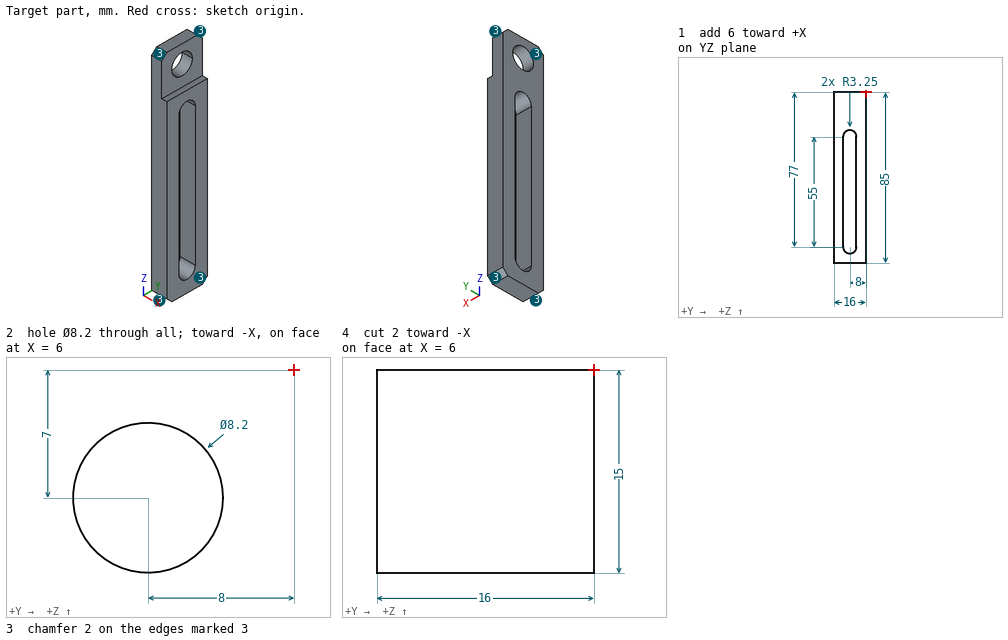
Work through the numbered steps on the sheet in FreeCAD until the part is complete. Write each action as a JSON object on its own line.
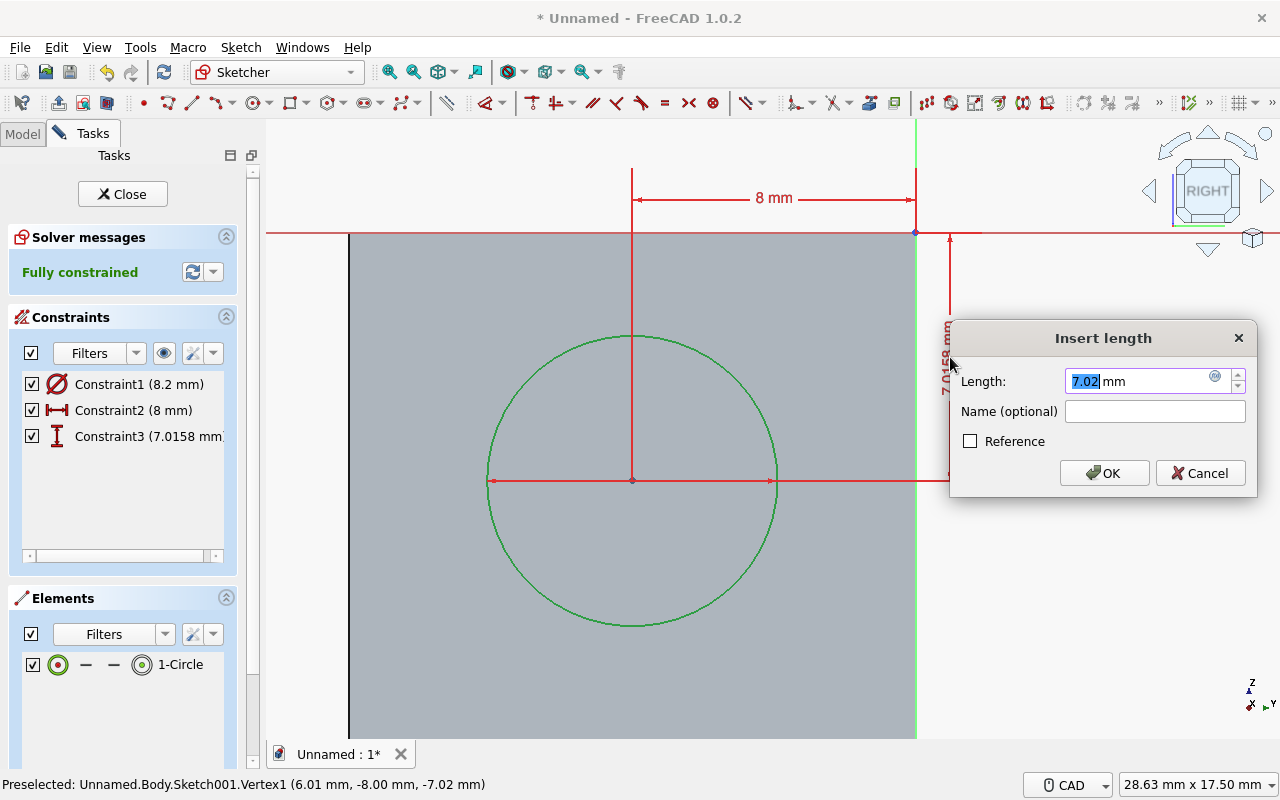
{"action": "type", "text": "7"}
{"action": "key", "text": "Return"}
{"action": "key", "text": "Escape"}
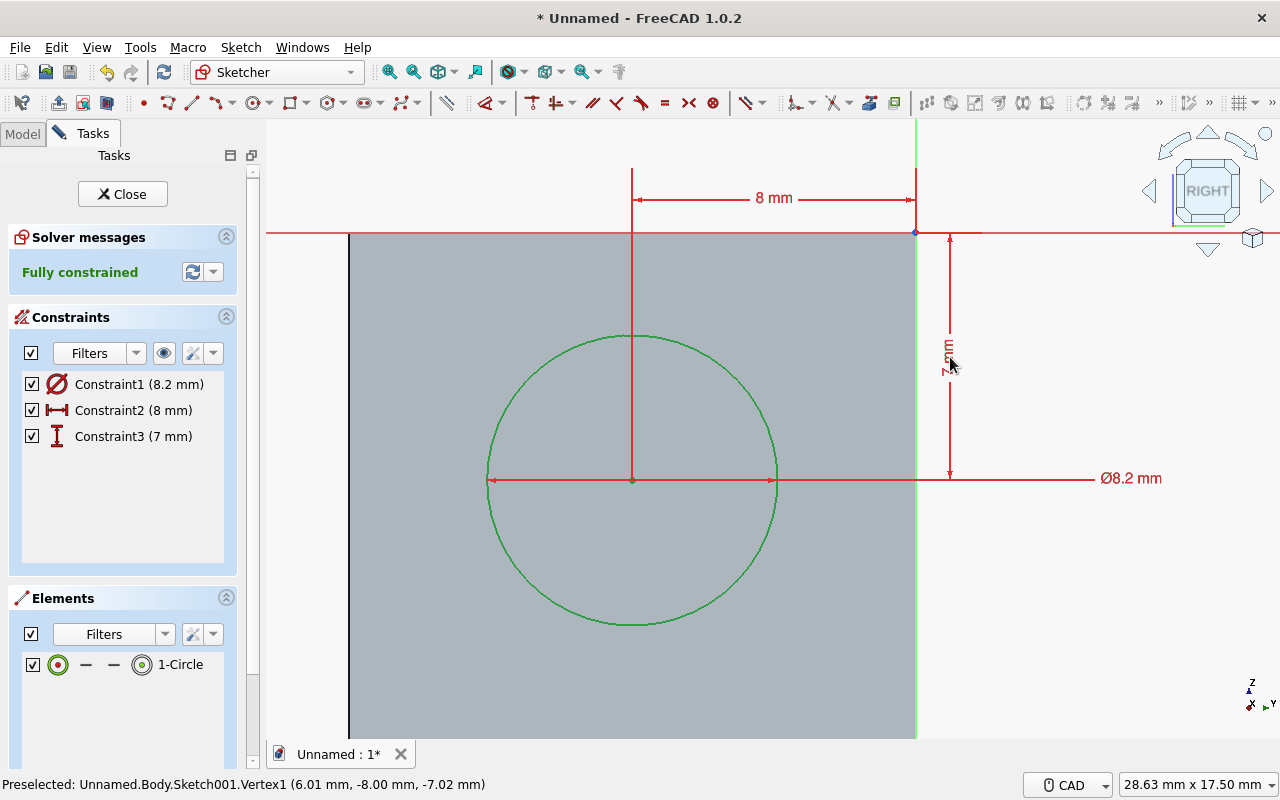
{"action": "left_click", "coordinate": [123, 194]}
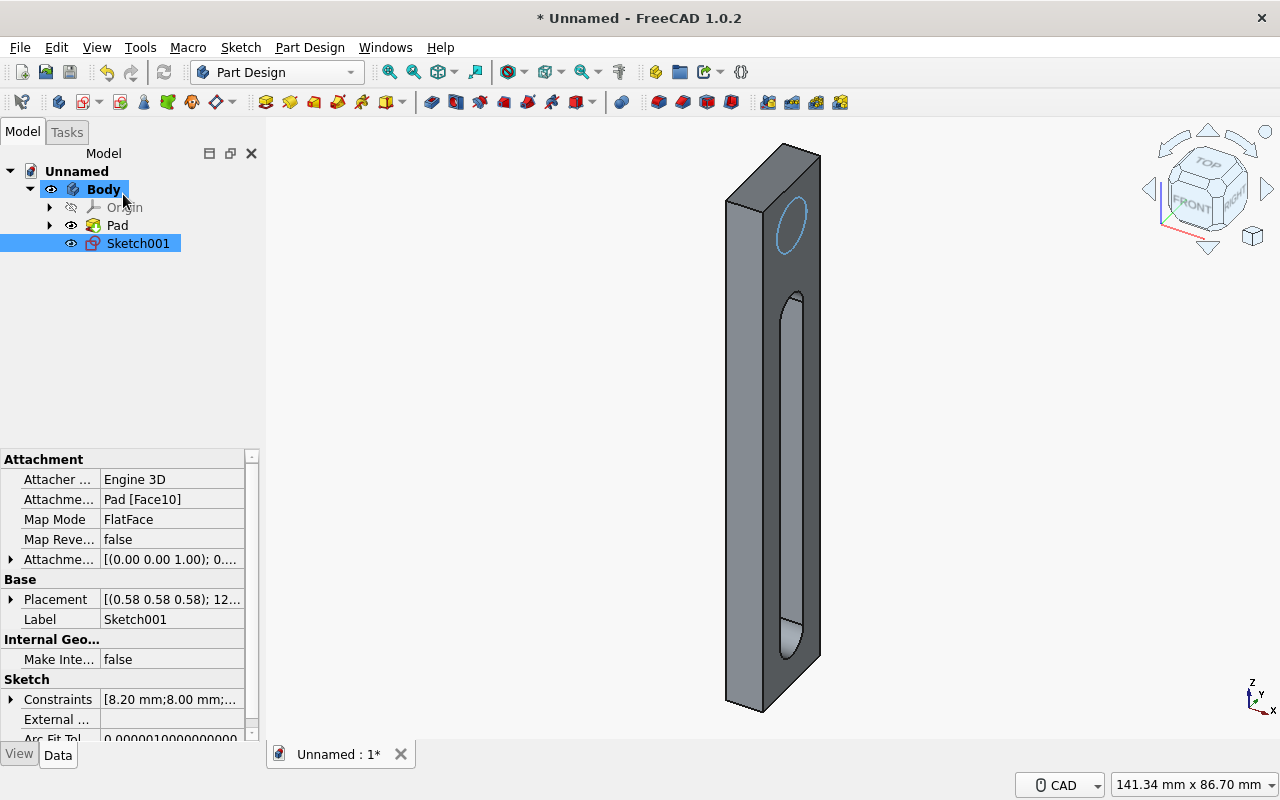
{"action": "left_click", "coordinate": [456, 102]}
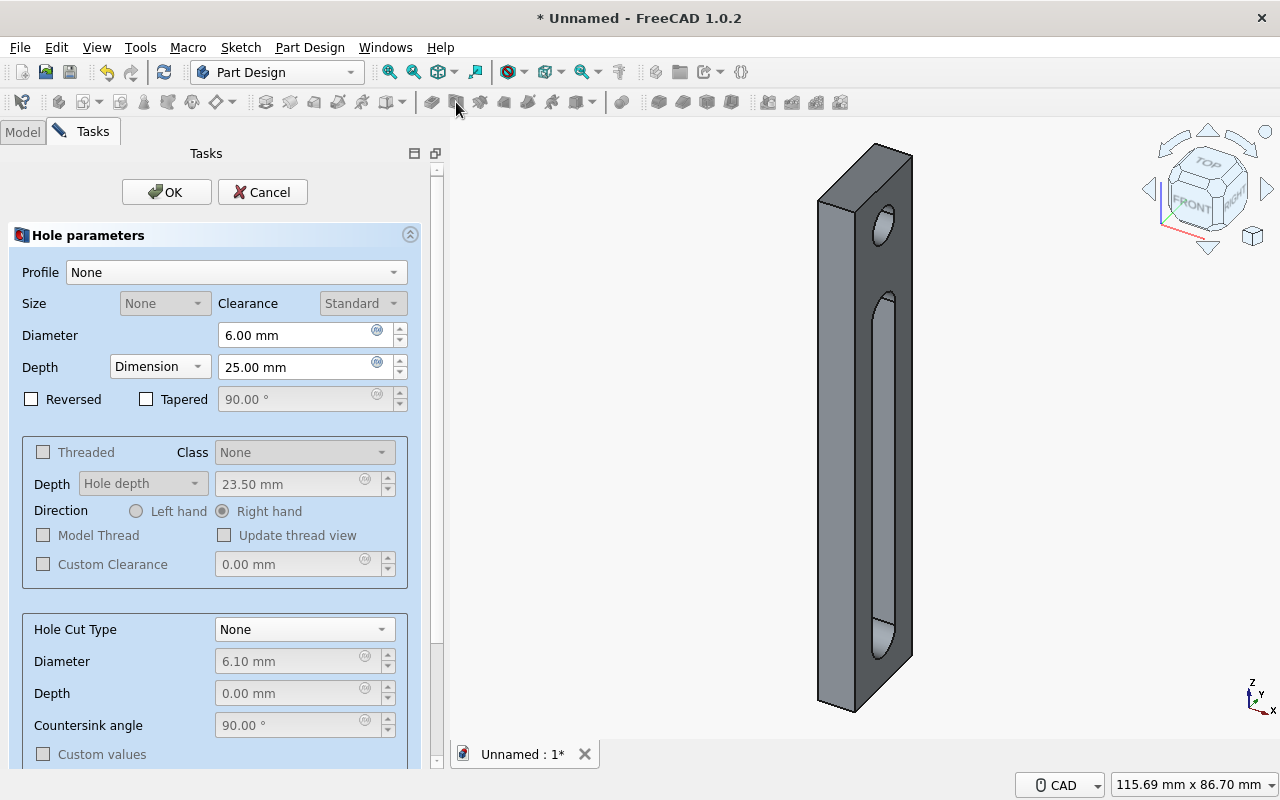
{"action": "triple_click", "coordinate": [305, 335]}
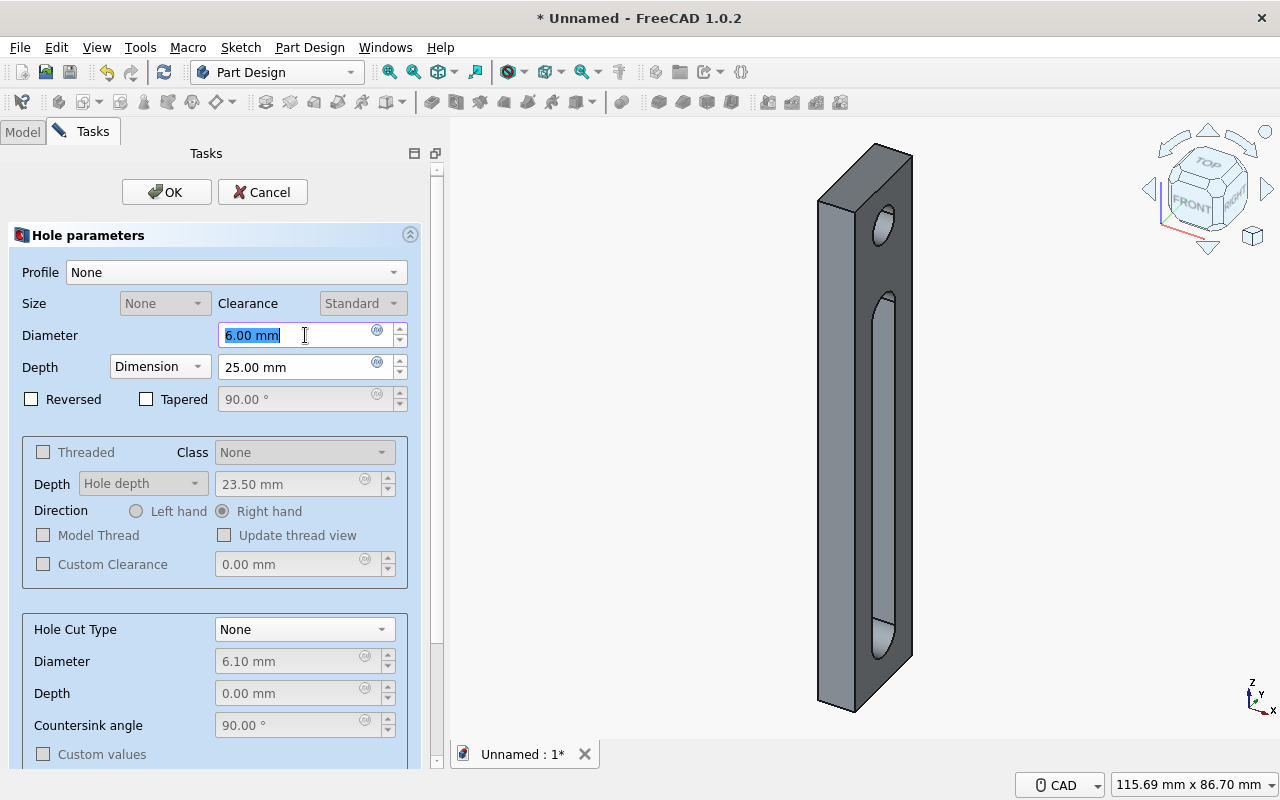
{"action": "type", "text": "8.2"}
{"action": "key", "text": "Tab"}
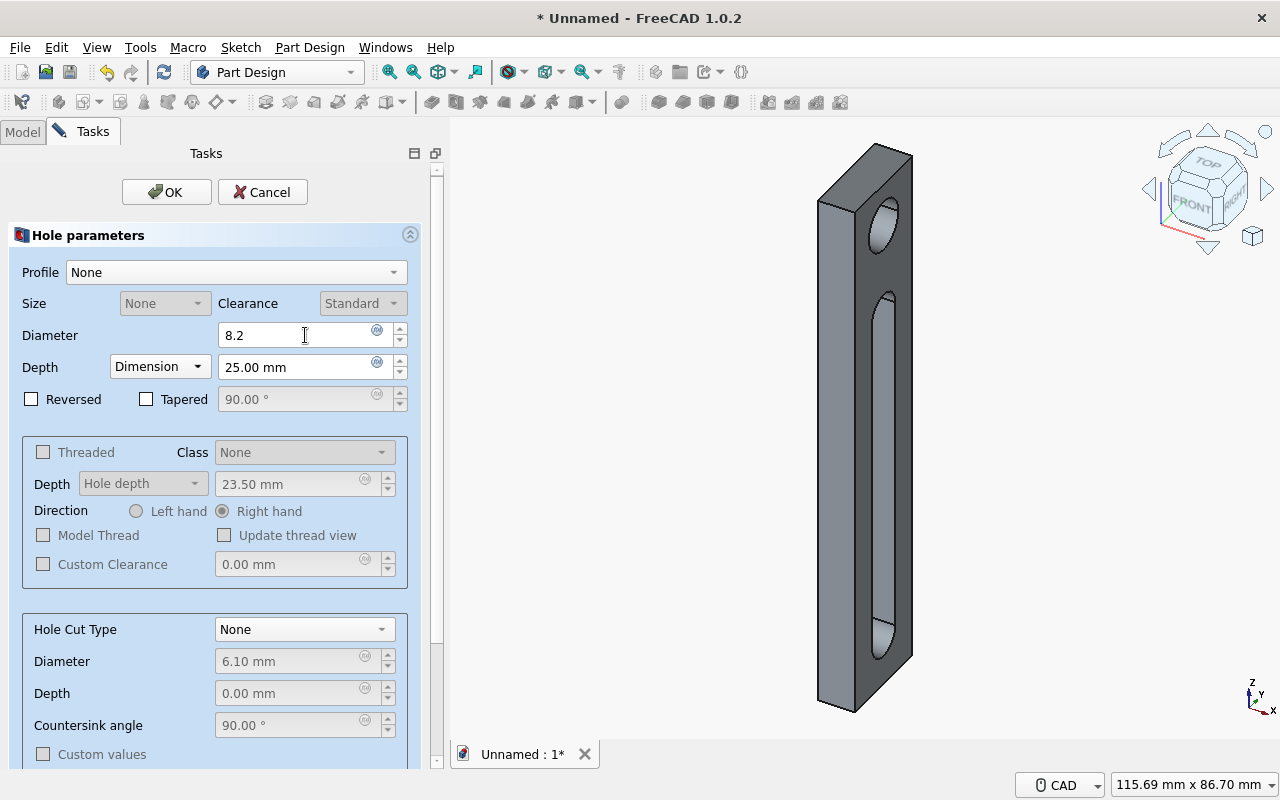
{"action": "left_click", "coordinate": [161, 366]}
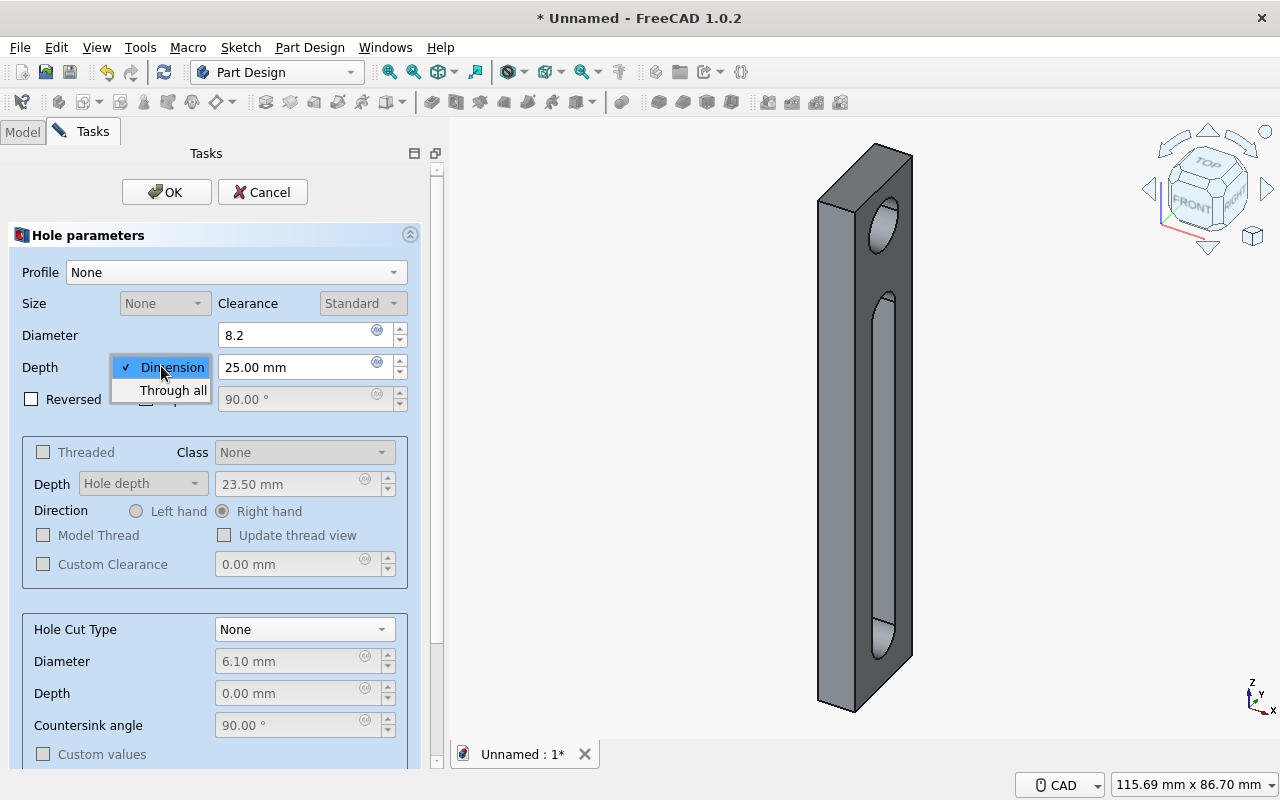
{"action": "left_click", "coordinate": [160, 390]}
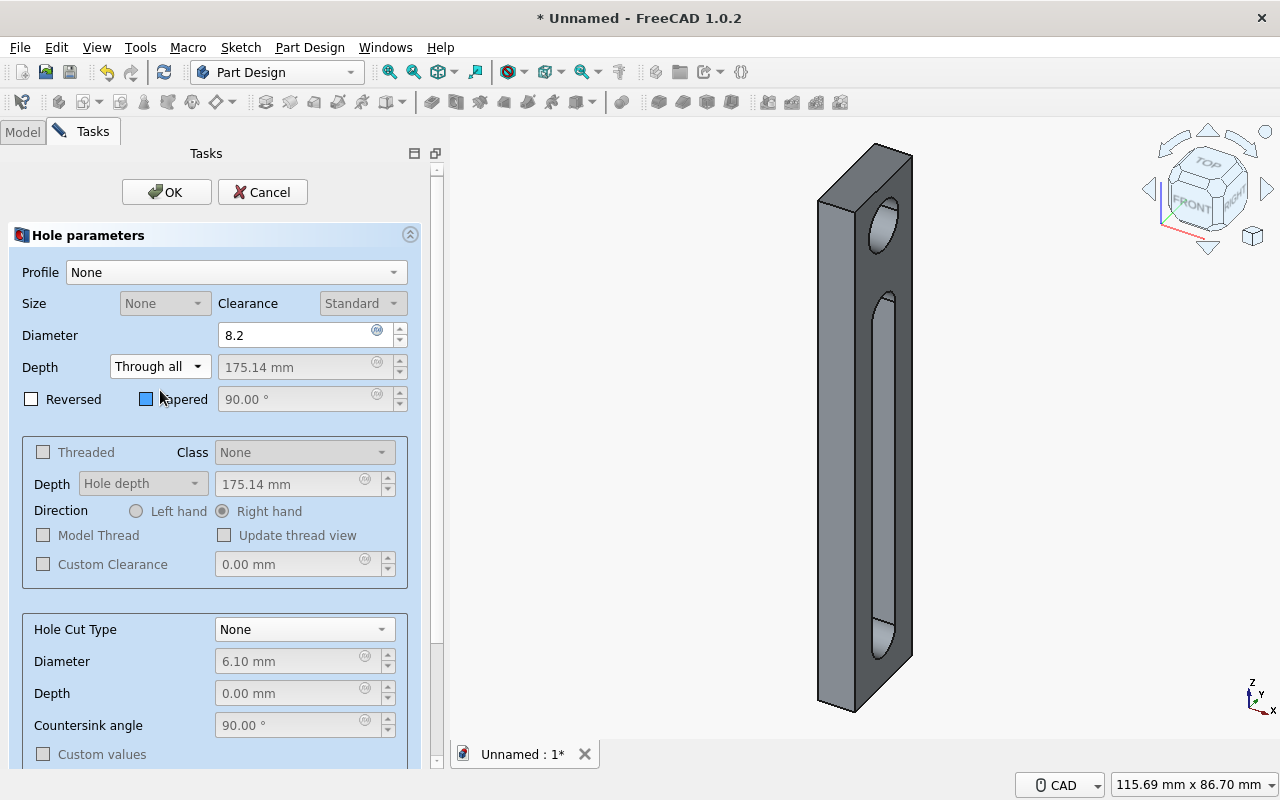
{"action": "left_click", "coordinate": [167, 192]}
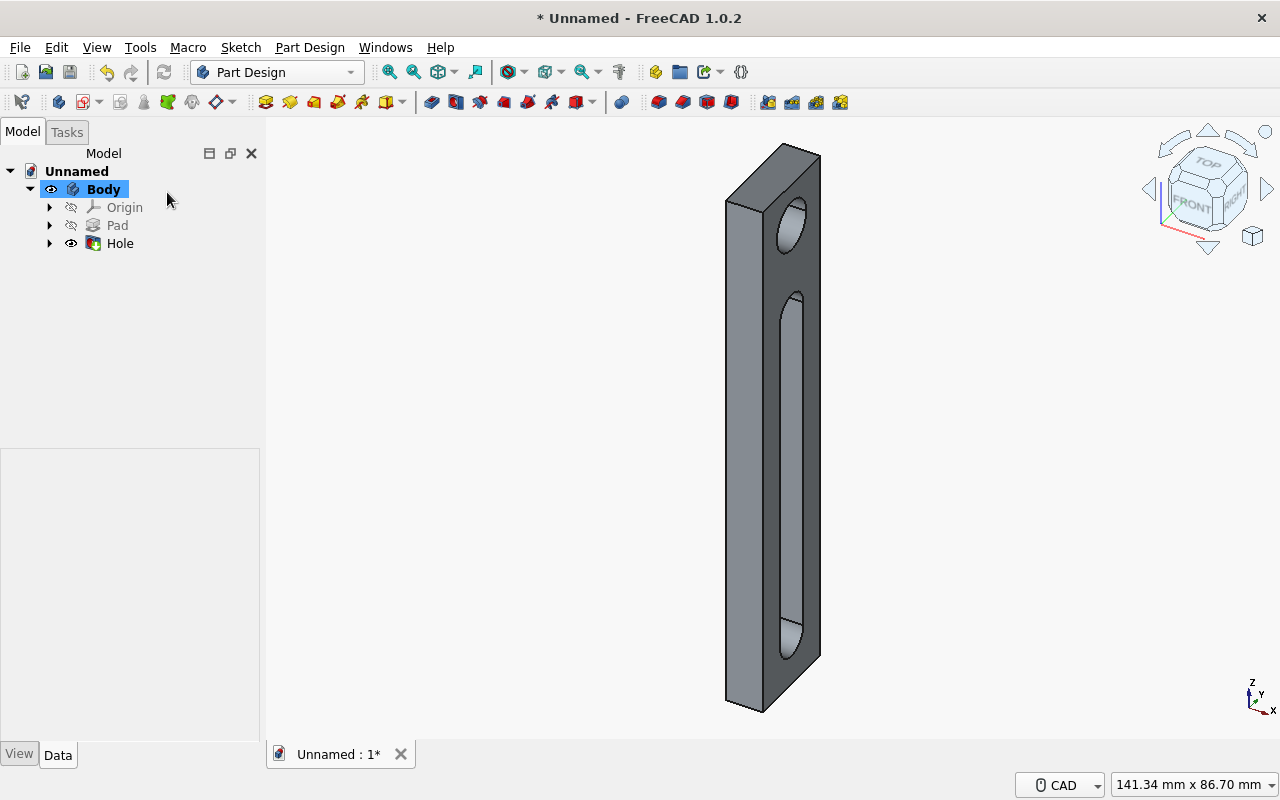
{"action": "left_click", "coordinate": [744, 206]}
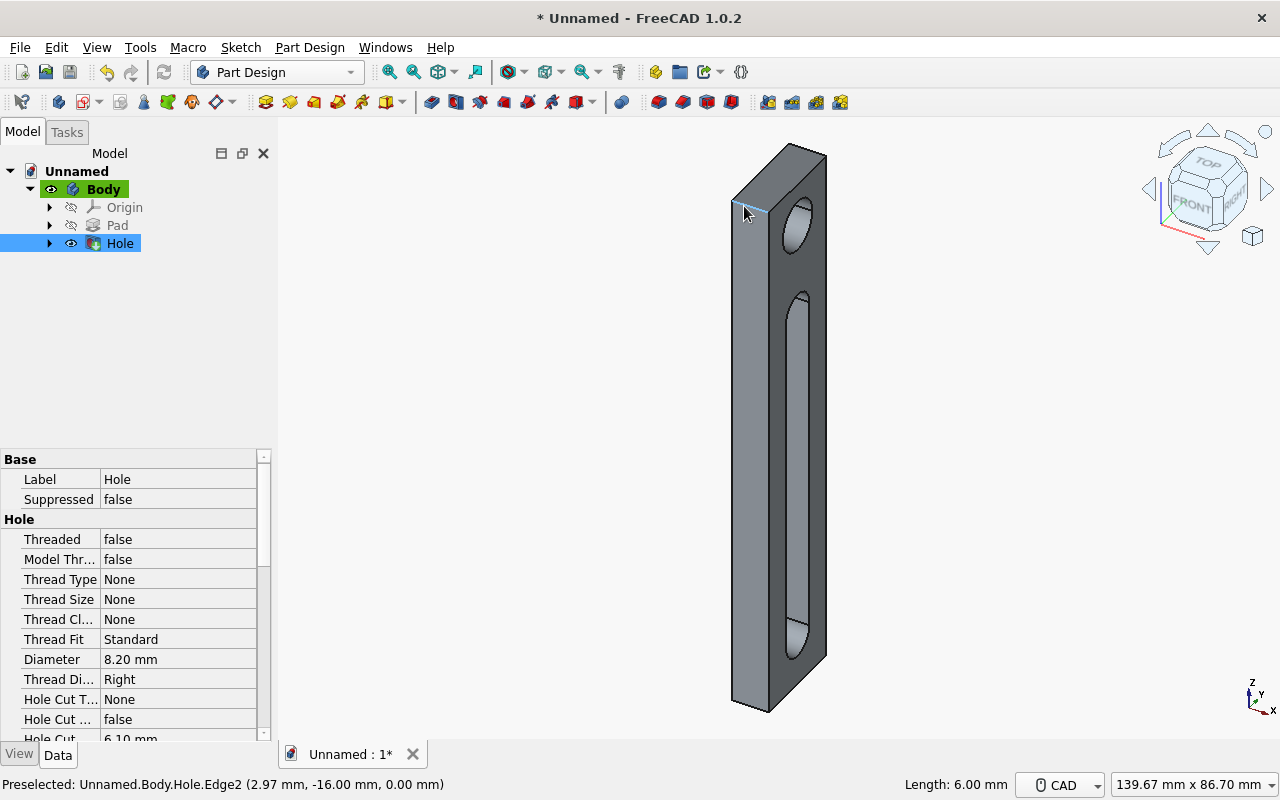
{"action": "key", "text": "0"}